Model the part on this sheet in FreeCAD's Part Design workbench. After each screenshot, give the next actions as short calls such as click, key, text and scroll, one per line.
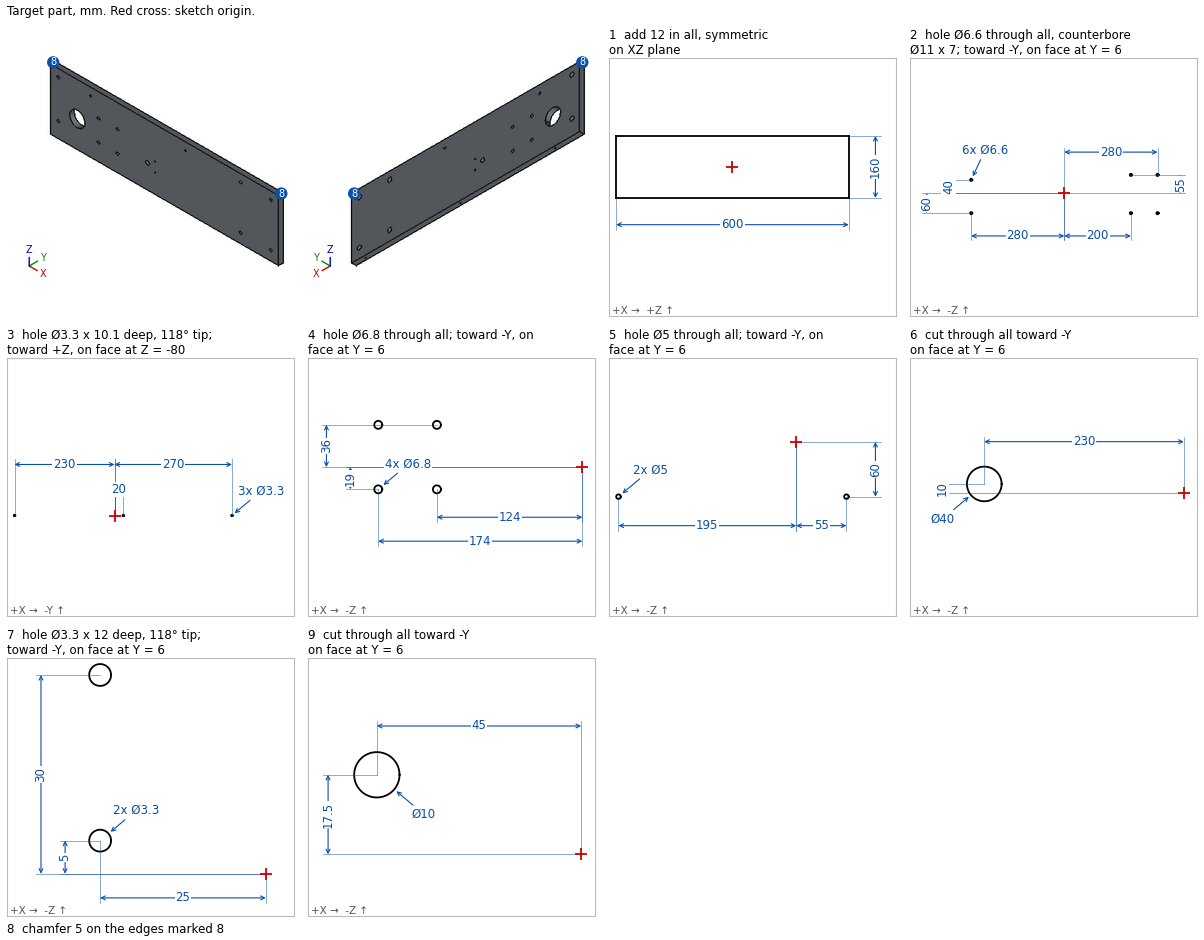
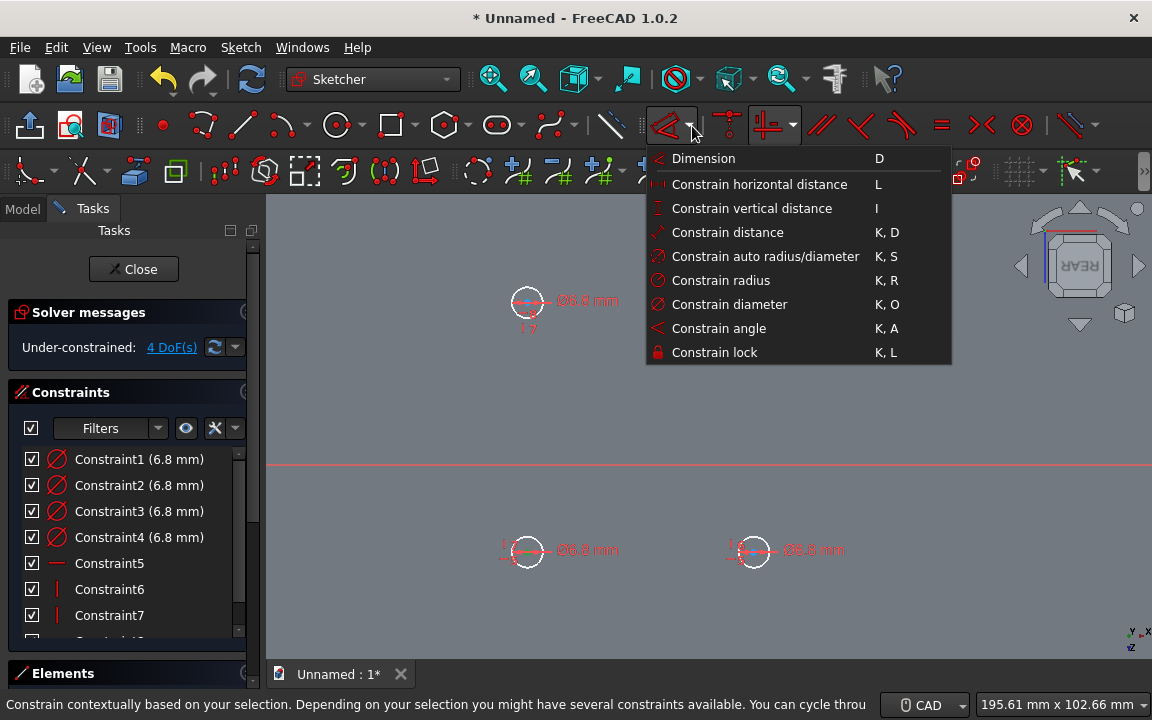
click(799, 208)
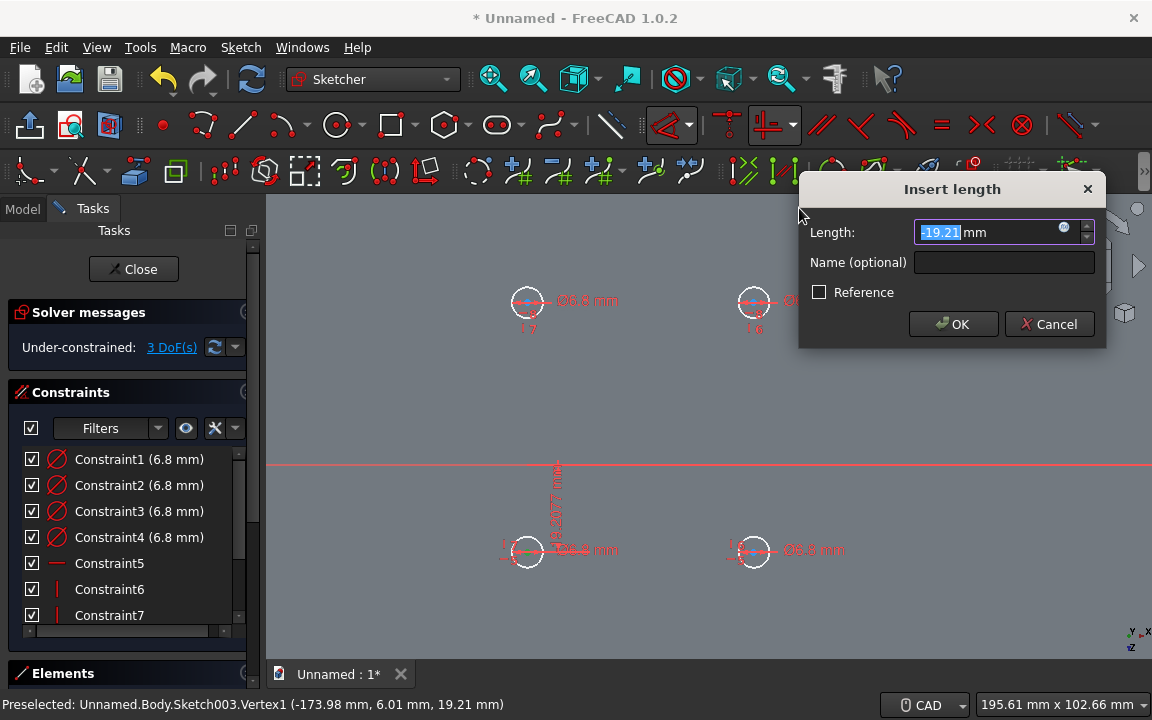
text(-19)
key(Return)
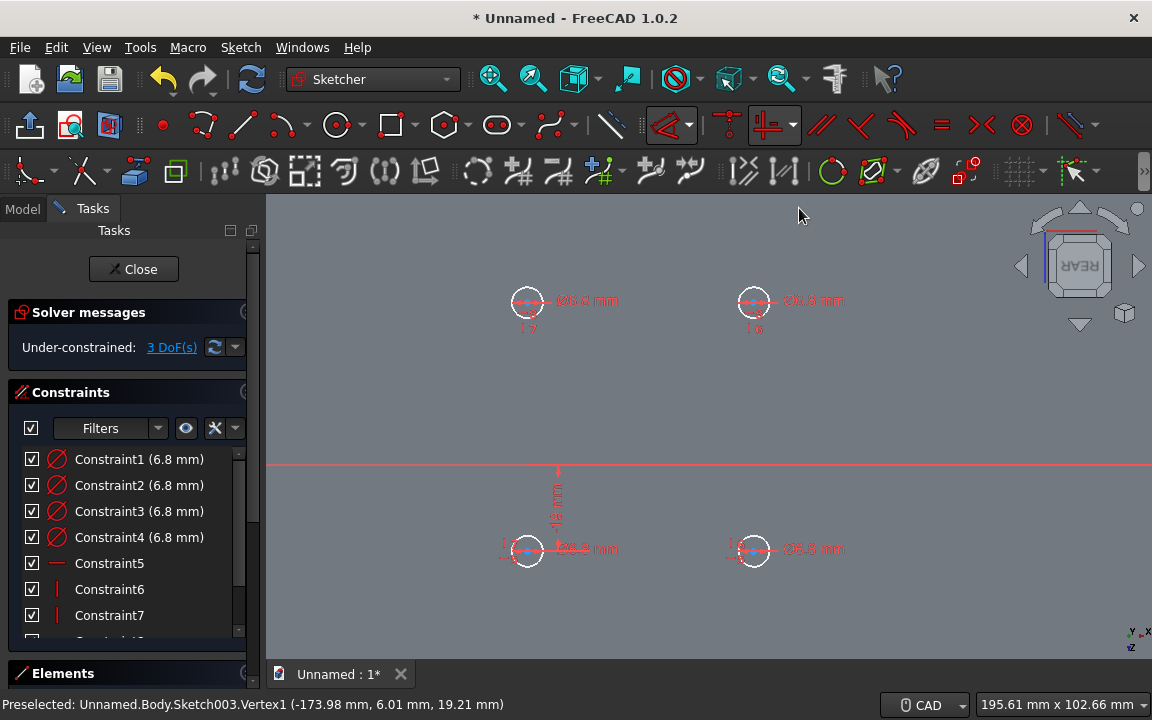
click(754, 303)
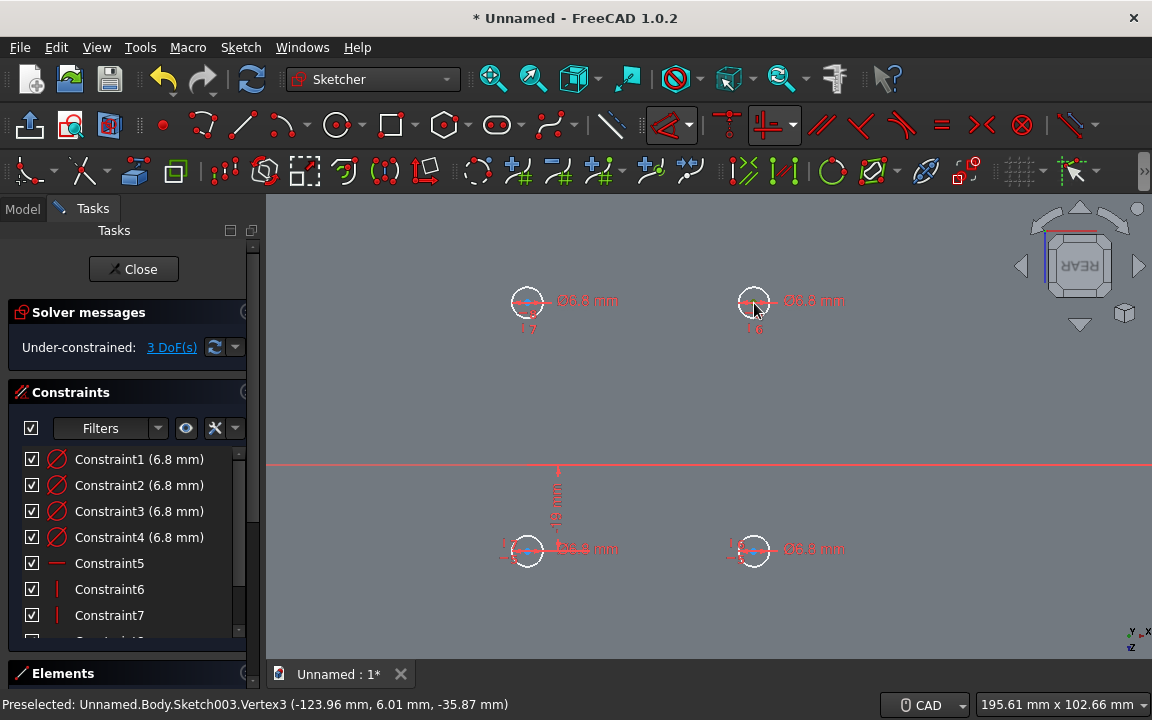
click(692, 126)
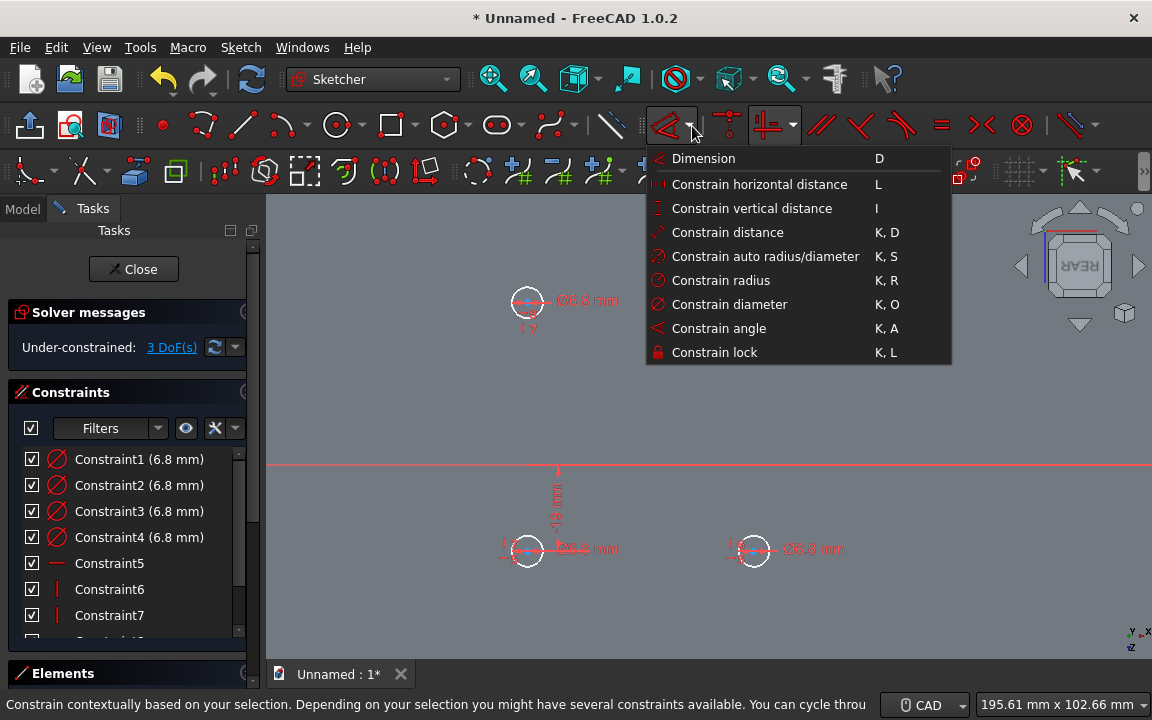
click(799, 208)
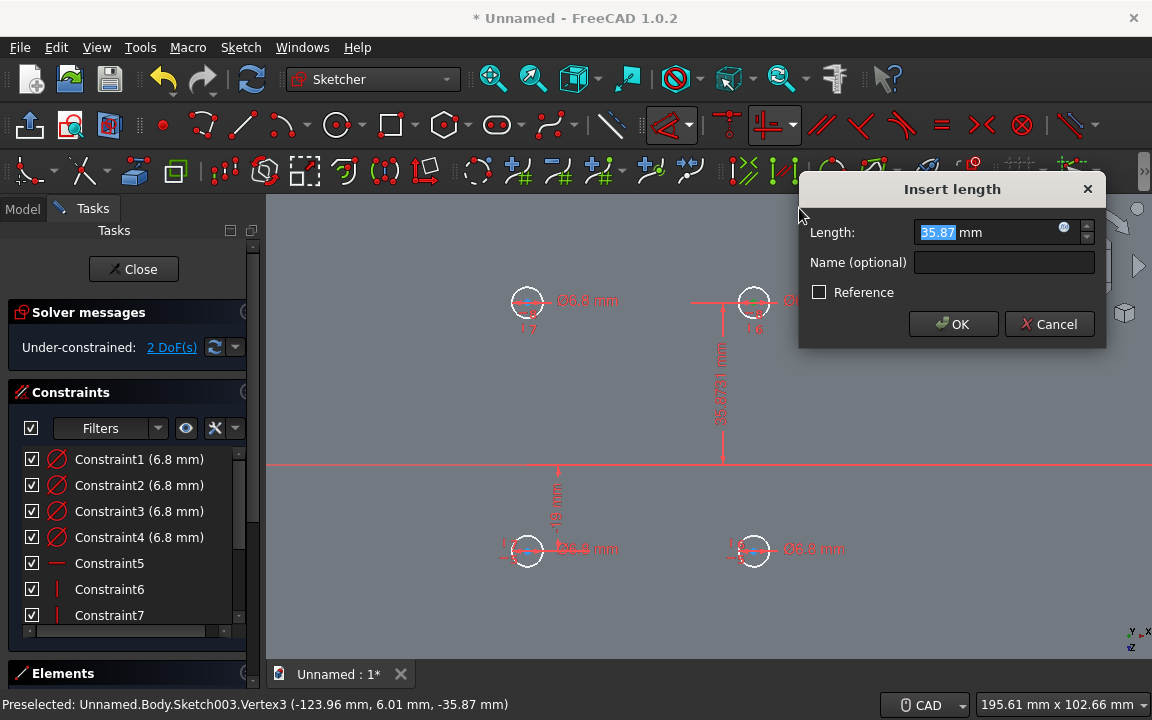
text(36)
key(Return)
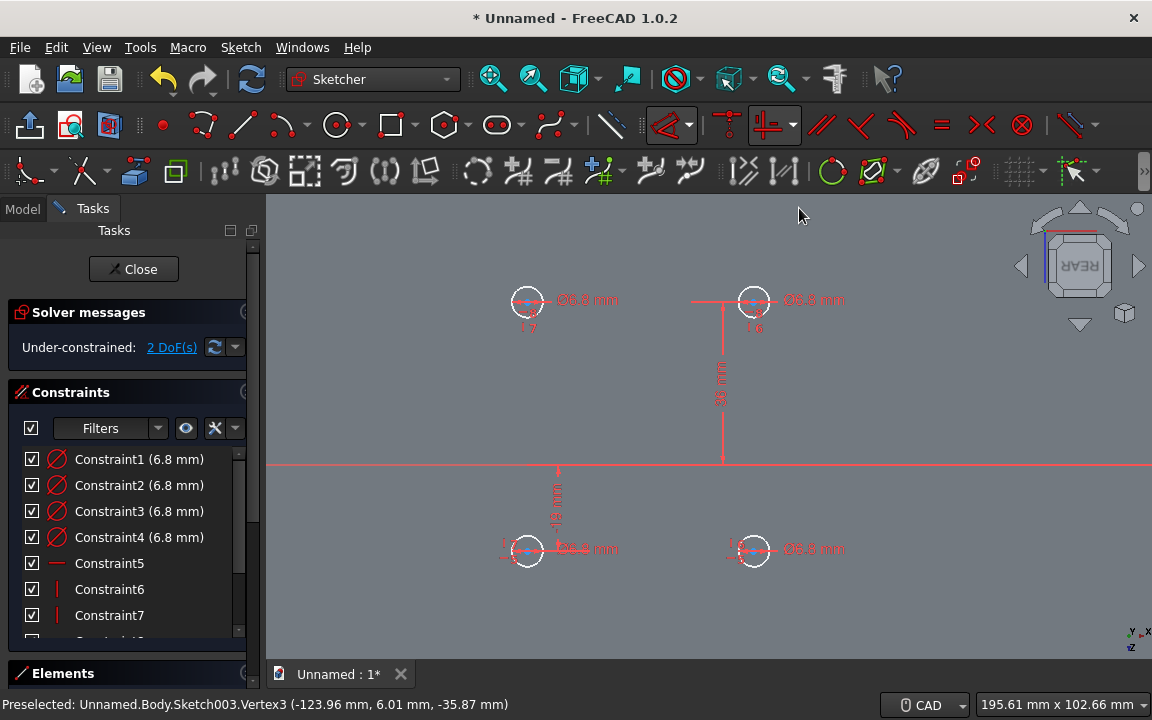
click(527, 551)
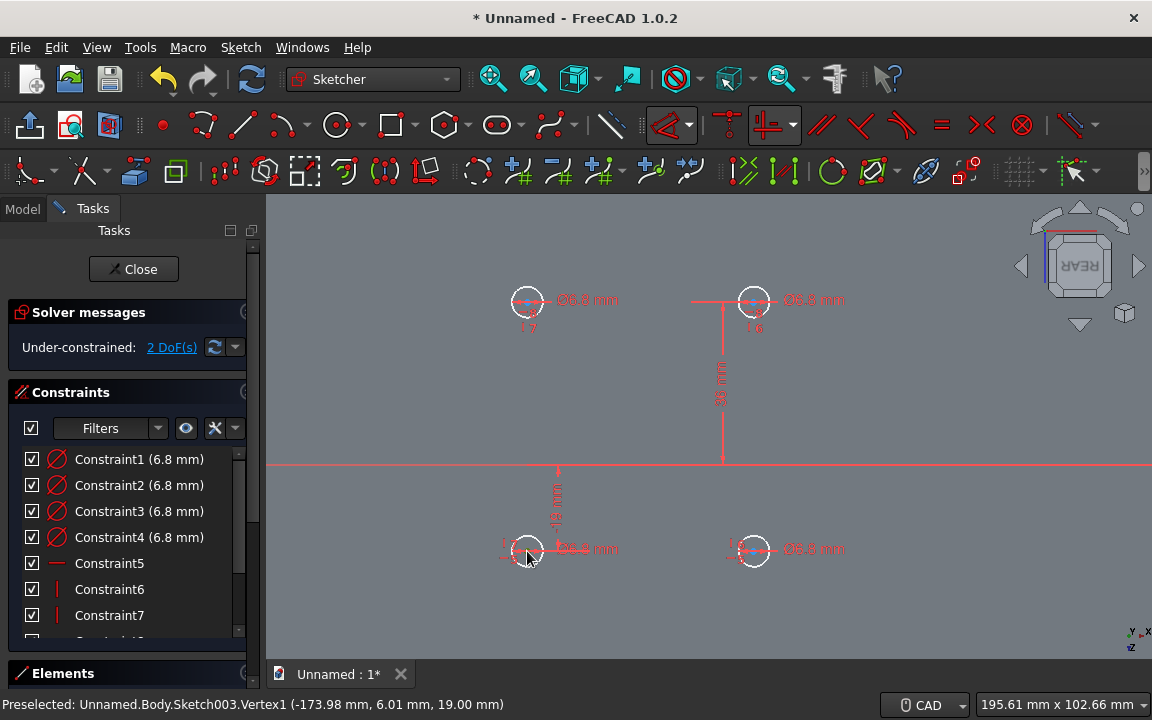
key(l)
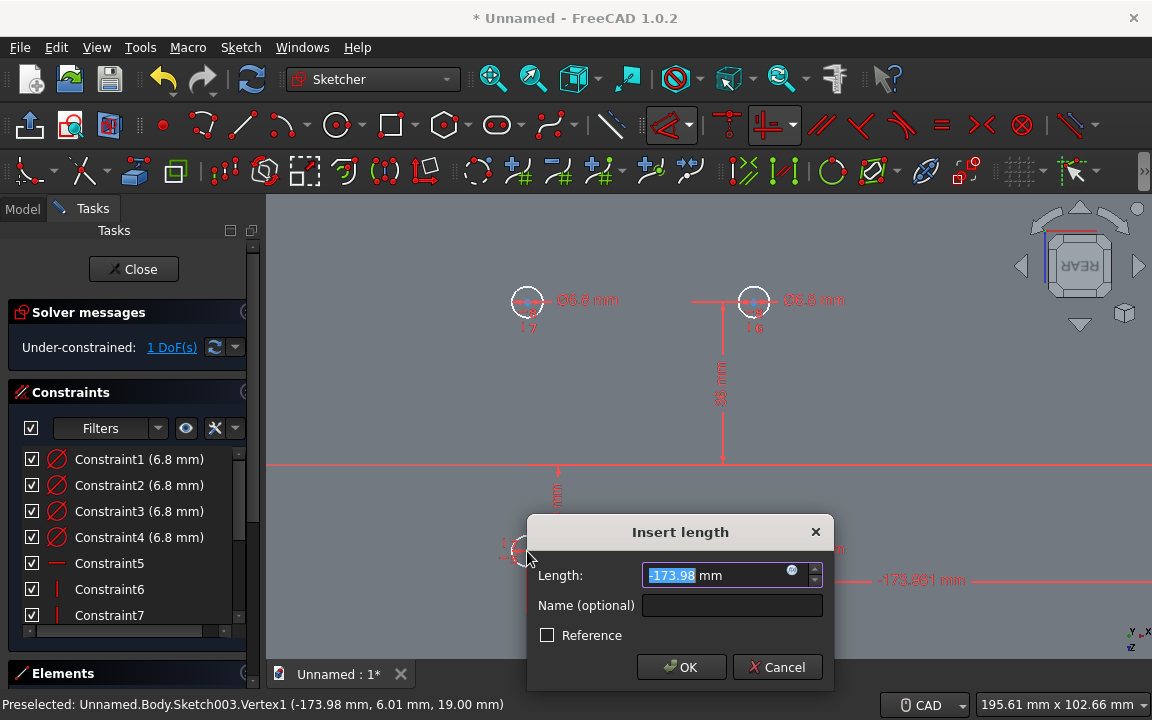
text(-174)
key(Return)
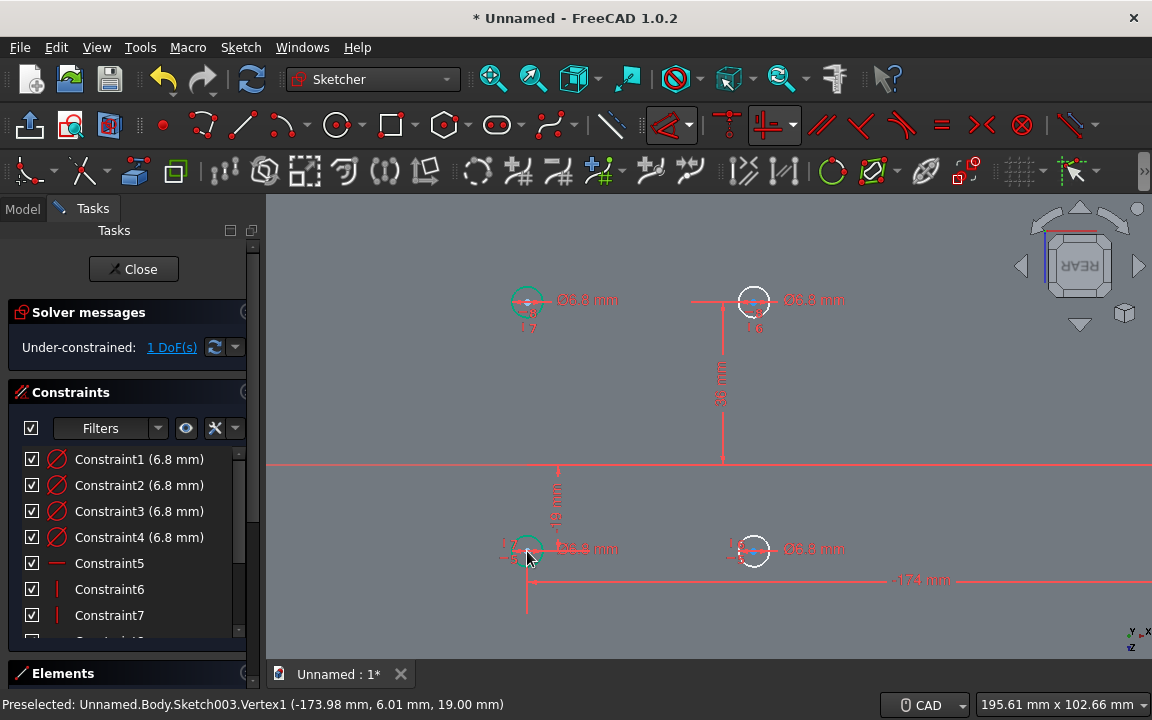
click(754, 551)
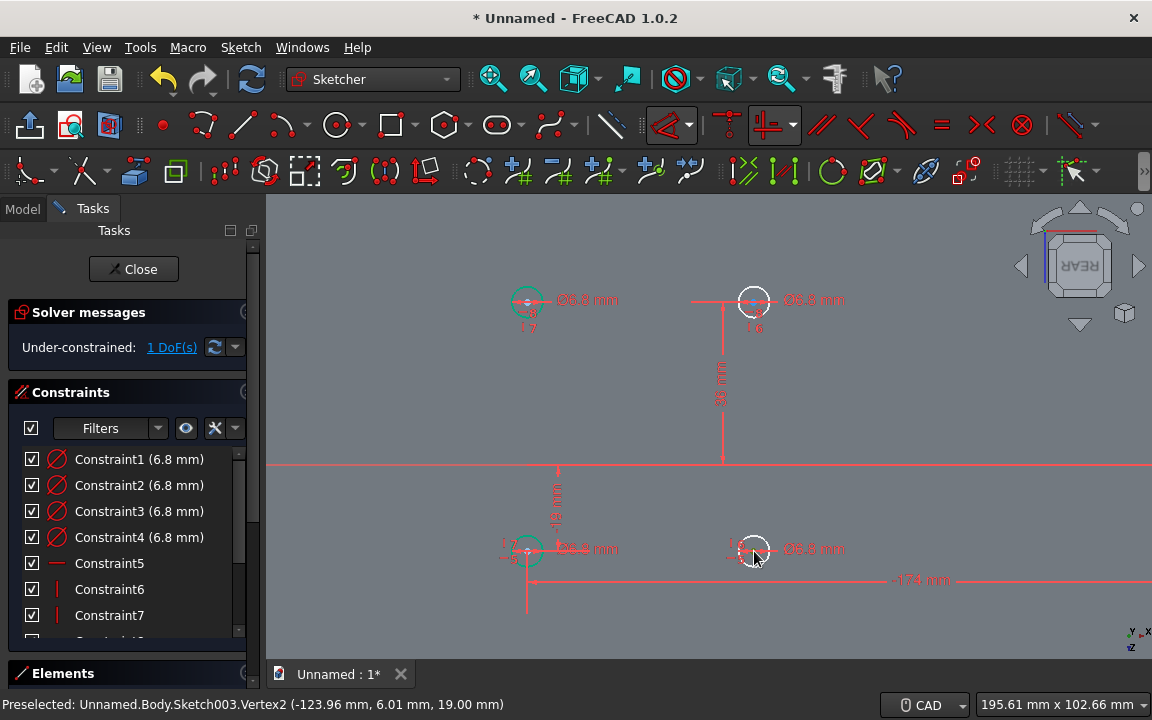
click(692, 126)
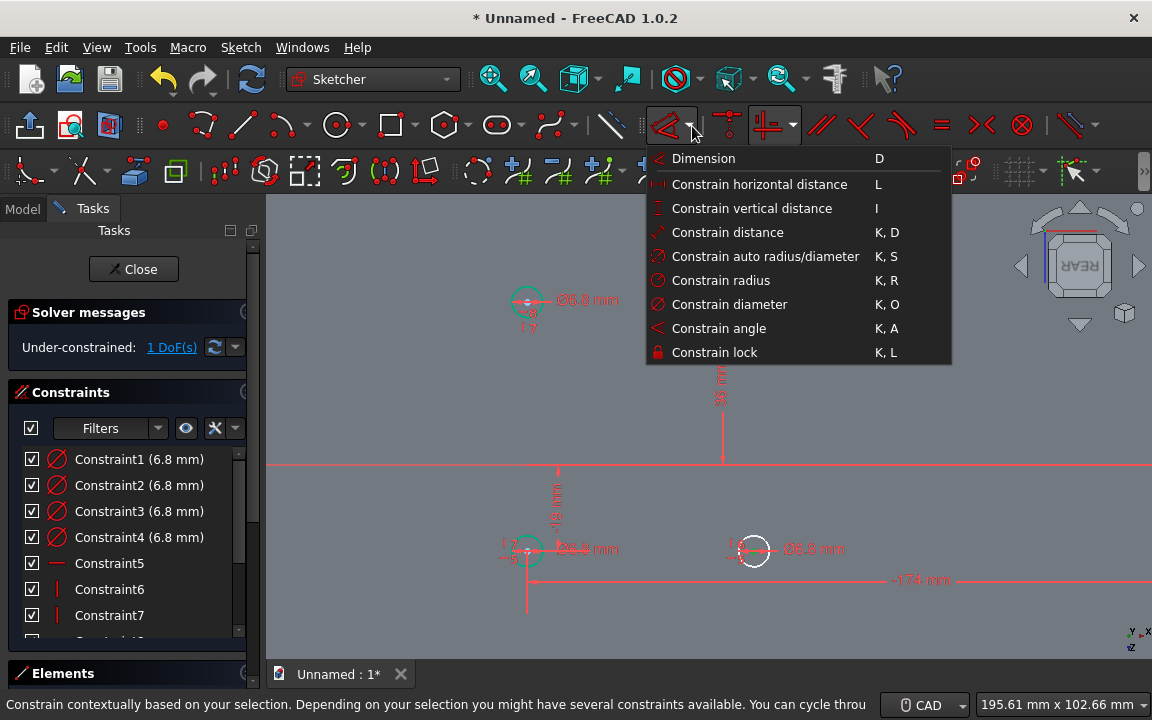
click(799, 184)